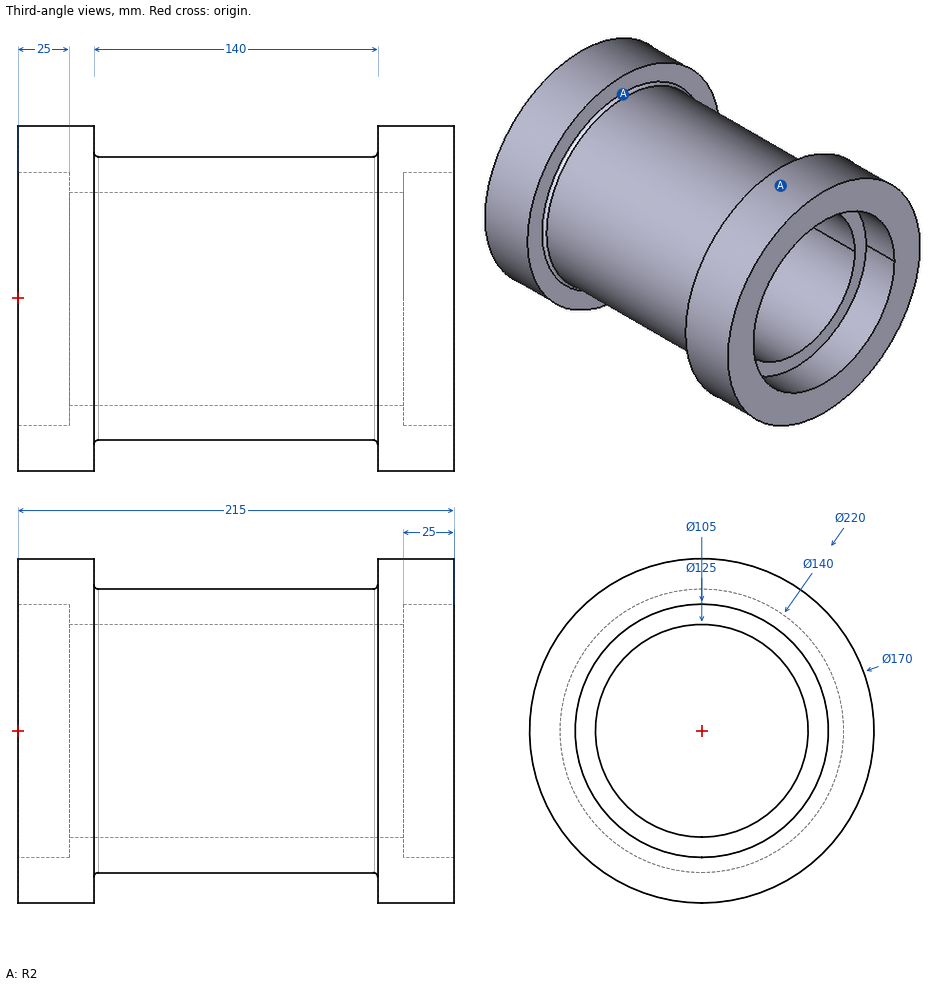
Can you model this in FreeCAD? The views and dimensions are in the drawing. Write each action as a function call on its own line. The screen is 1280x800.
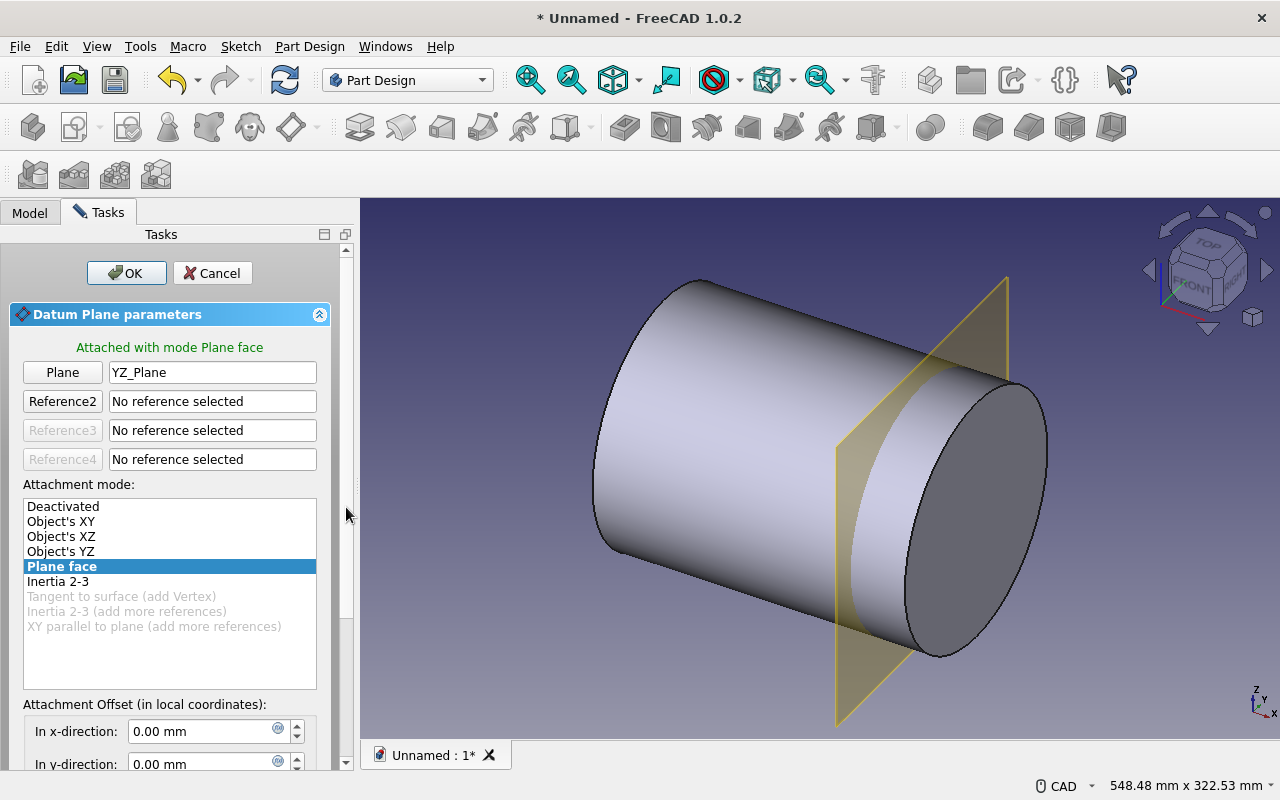
click(127, 273)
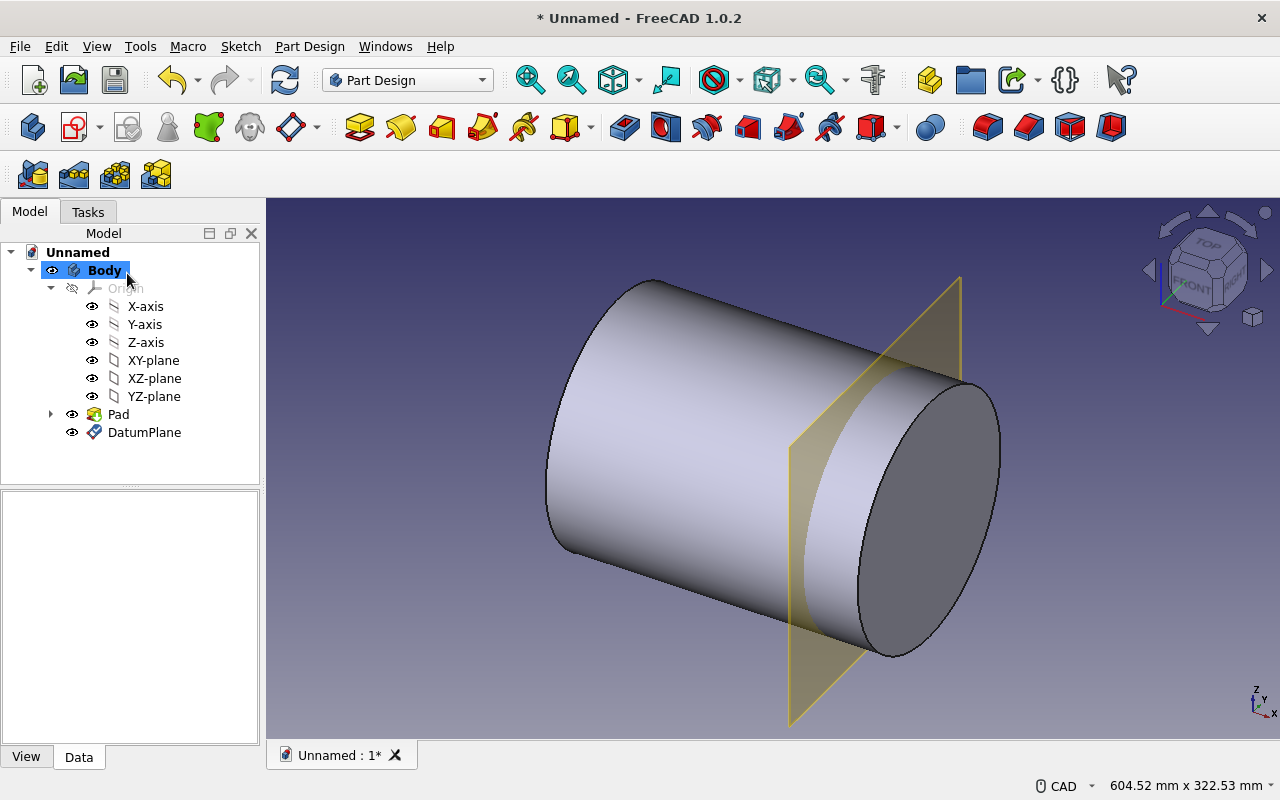
click(117, 432)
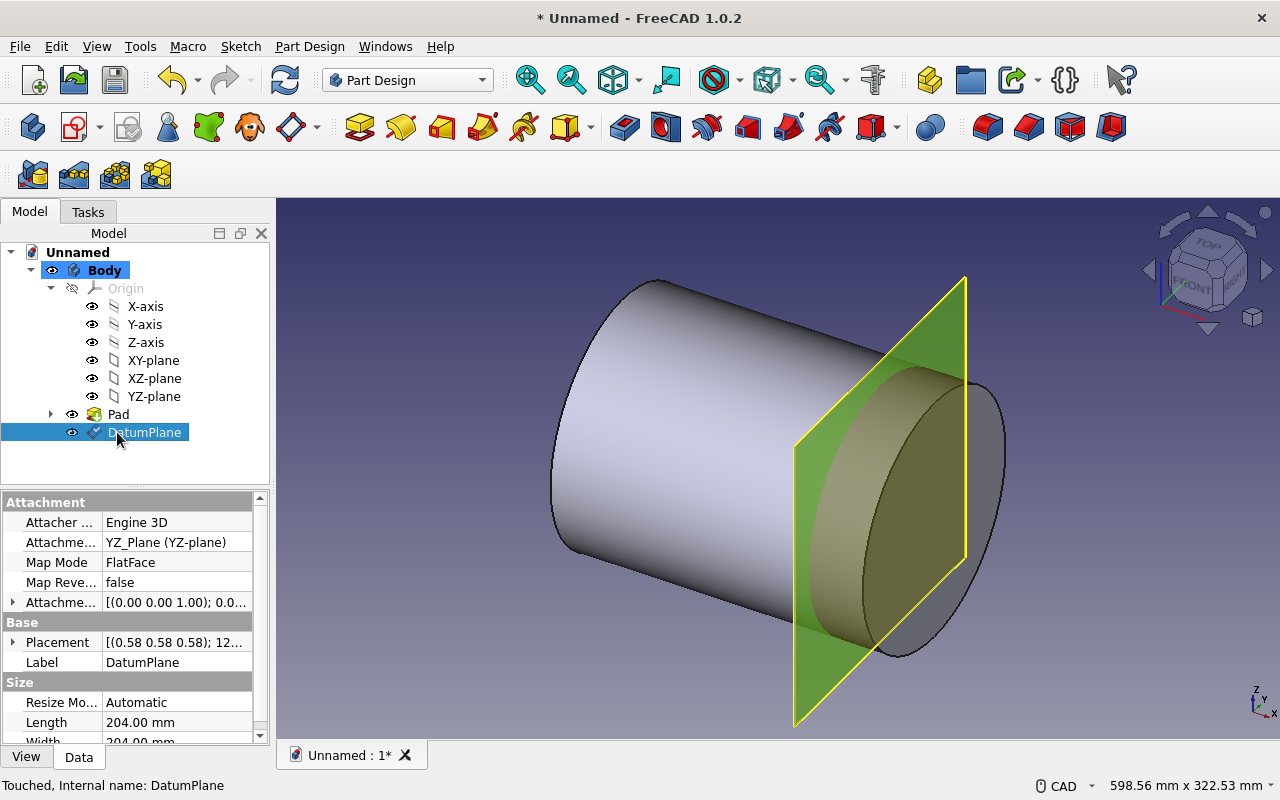
click(74, 128)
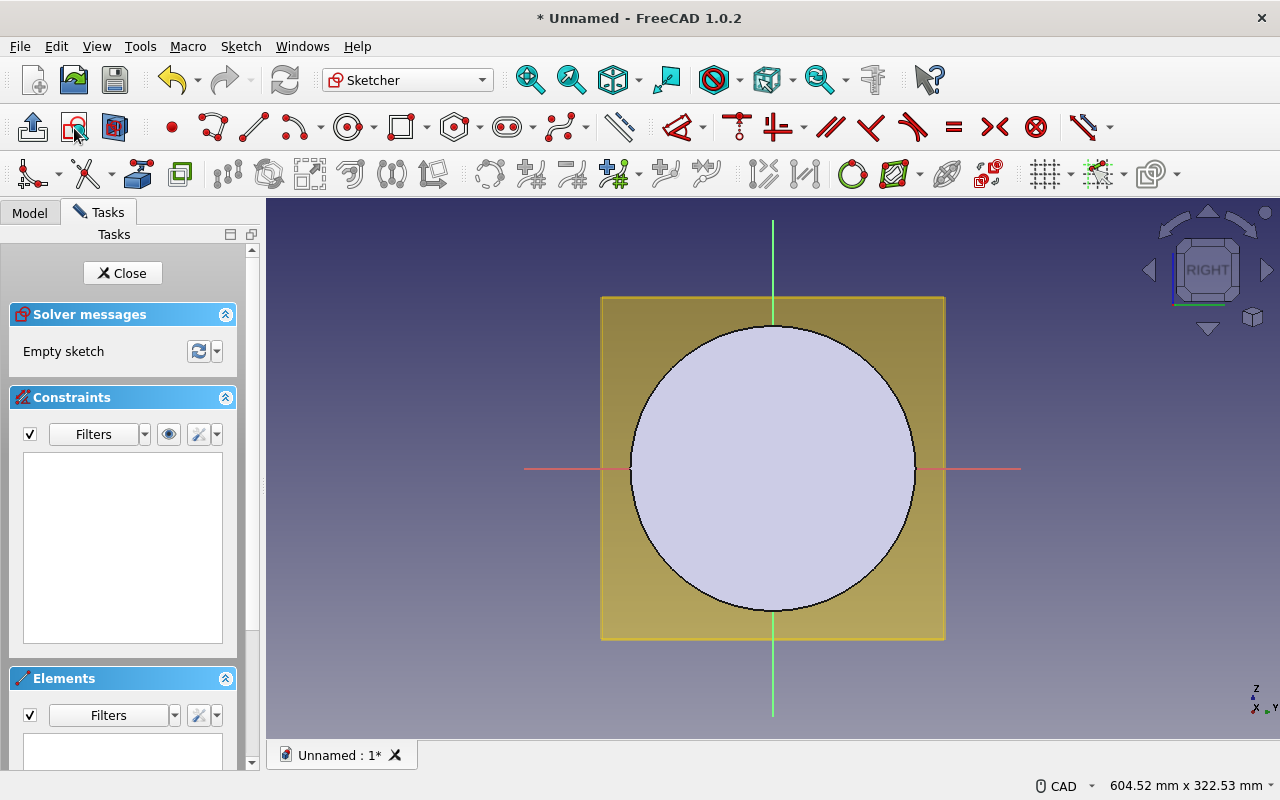
key(q)
key(s)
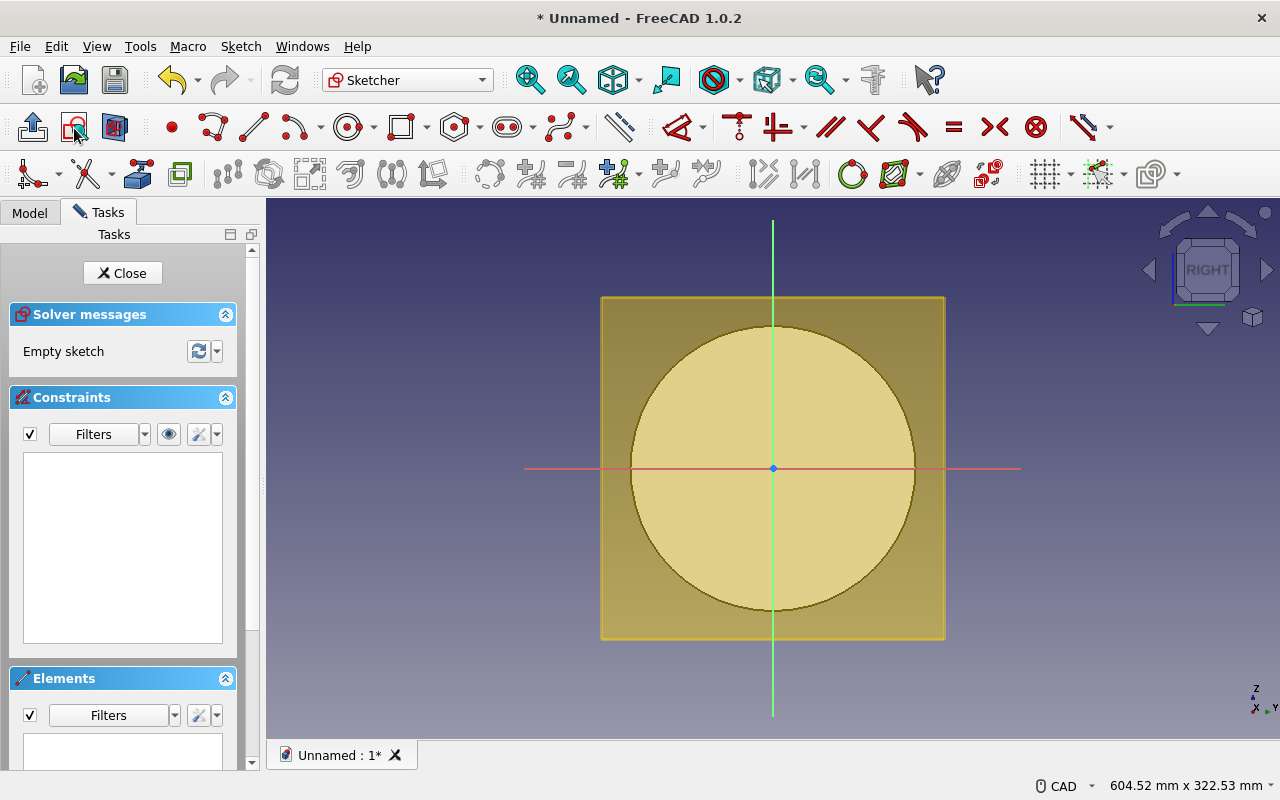
key(g)
key(c)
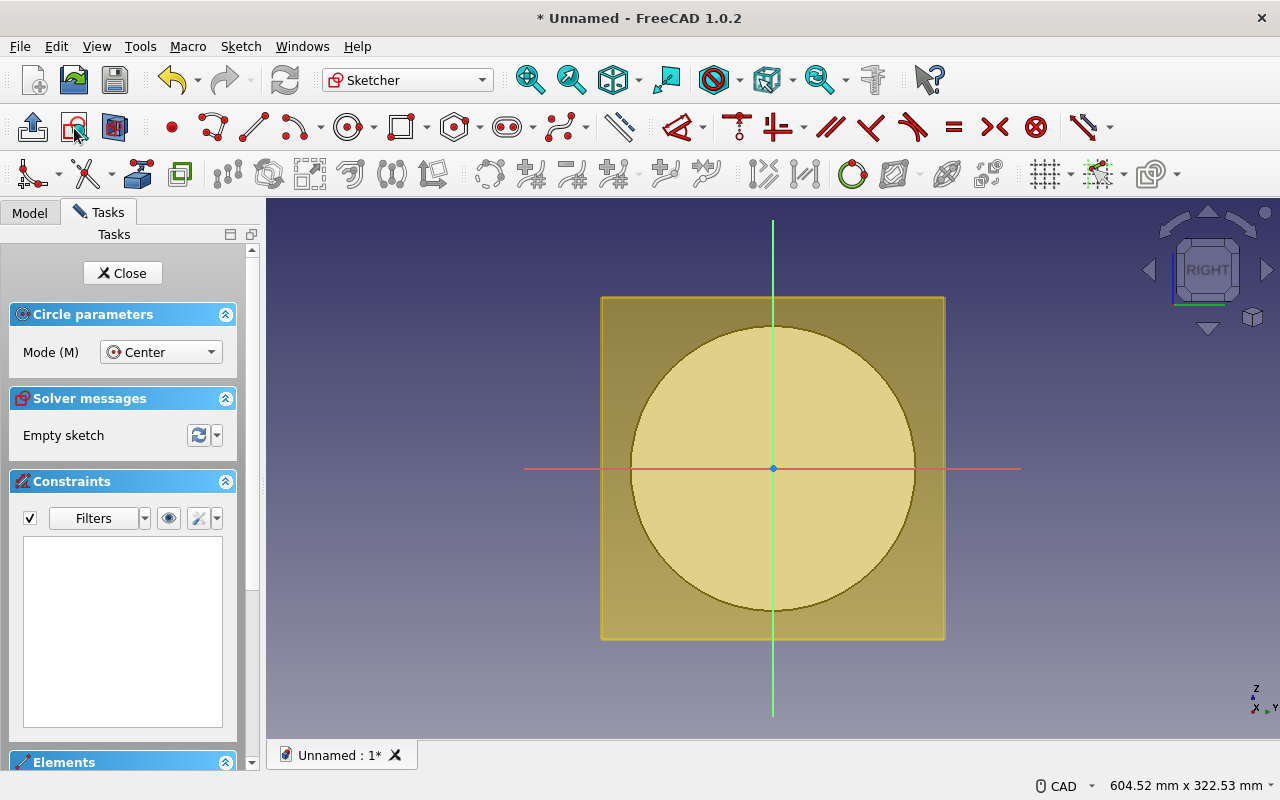
click(773, 468)
move(903, 338)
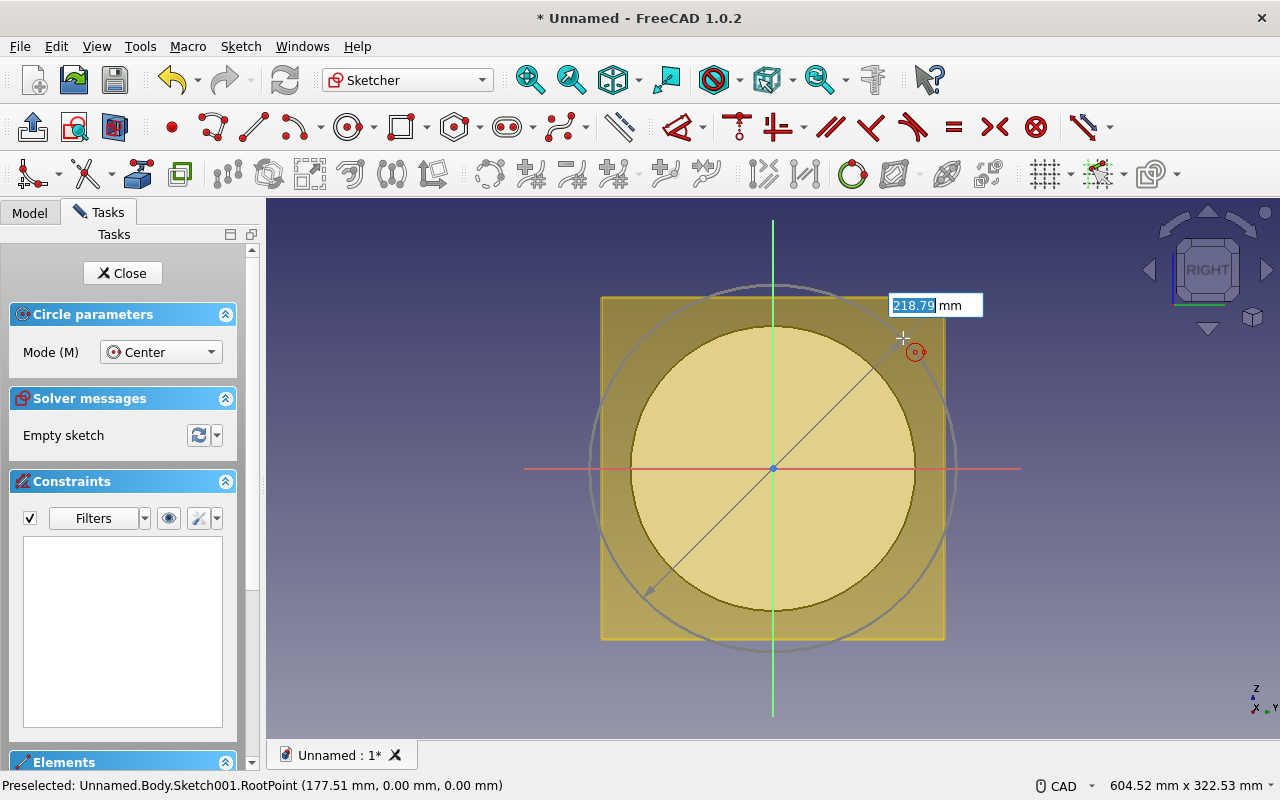
text(220)
key(Return)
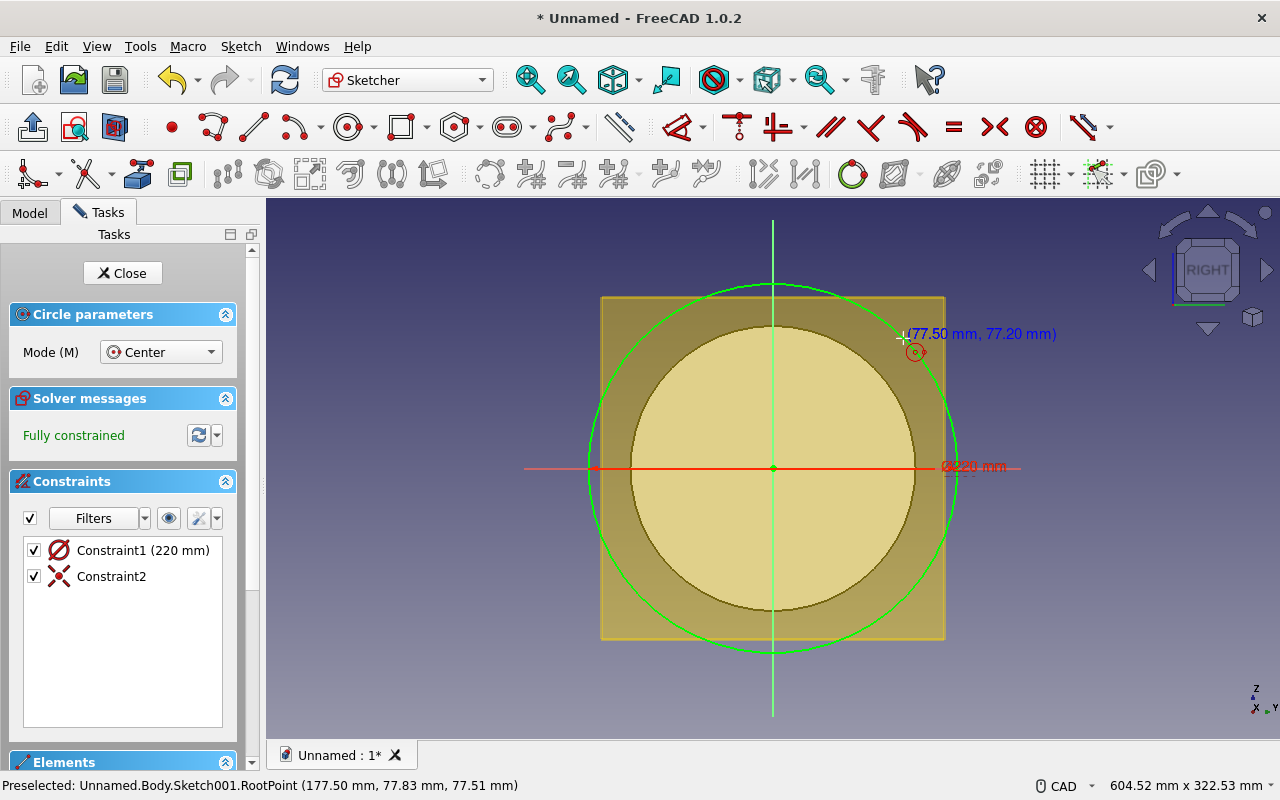
click(773, 468)
move(856, 385)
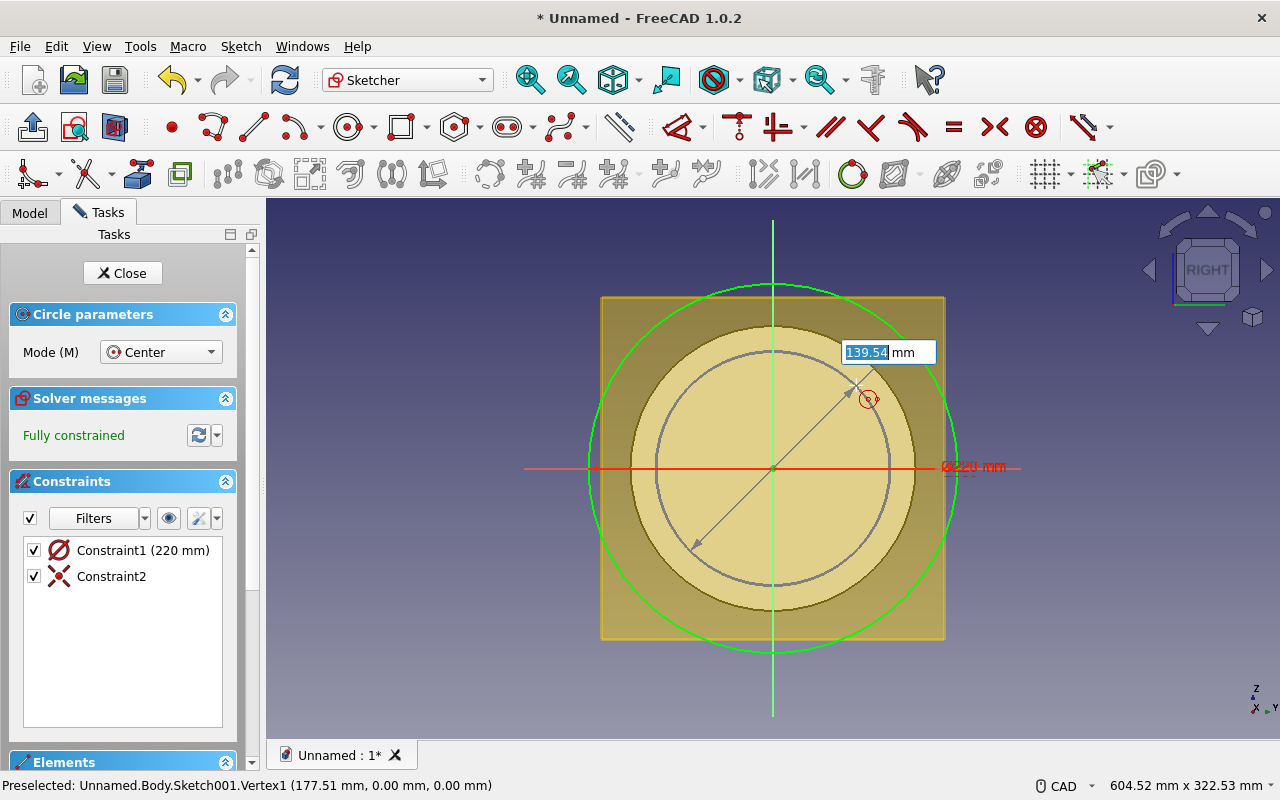
text(140)
key(Return)
key(Escape)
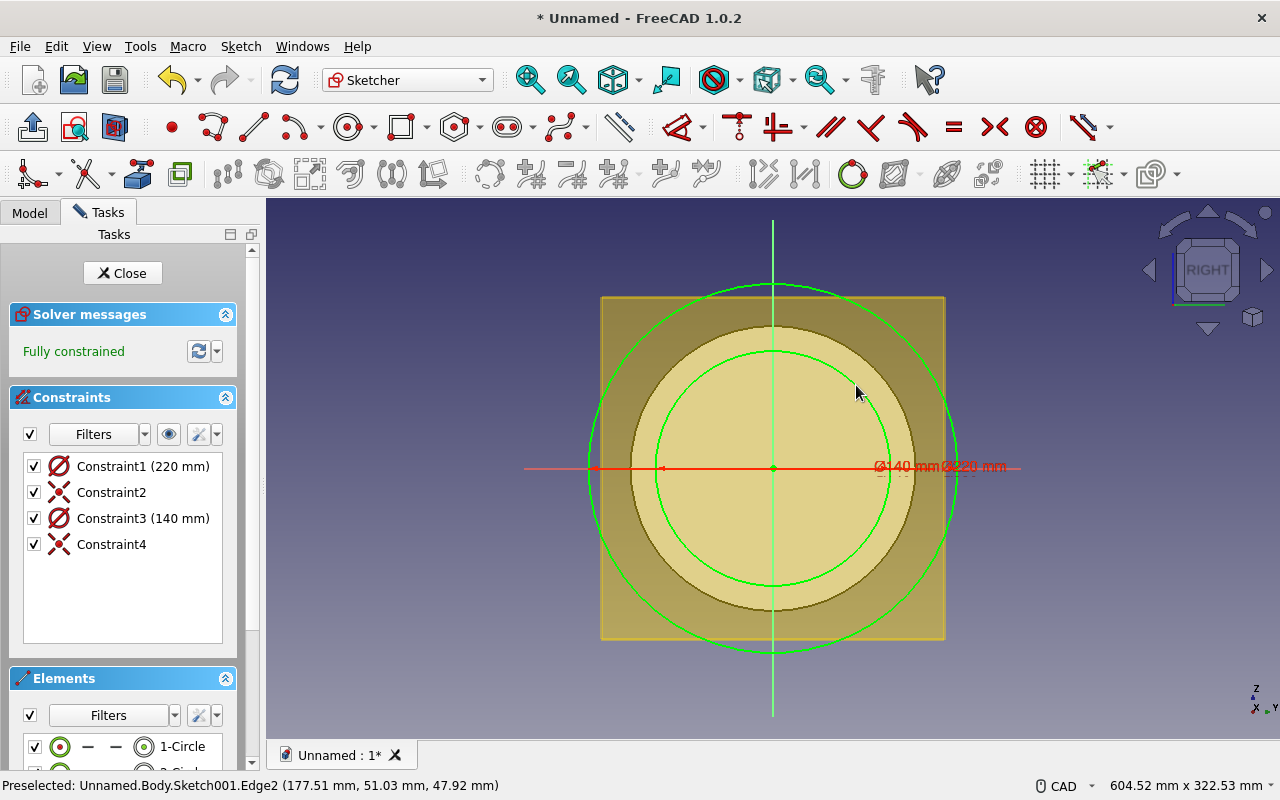
click(123, 273)